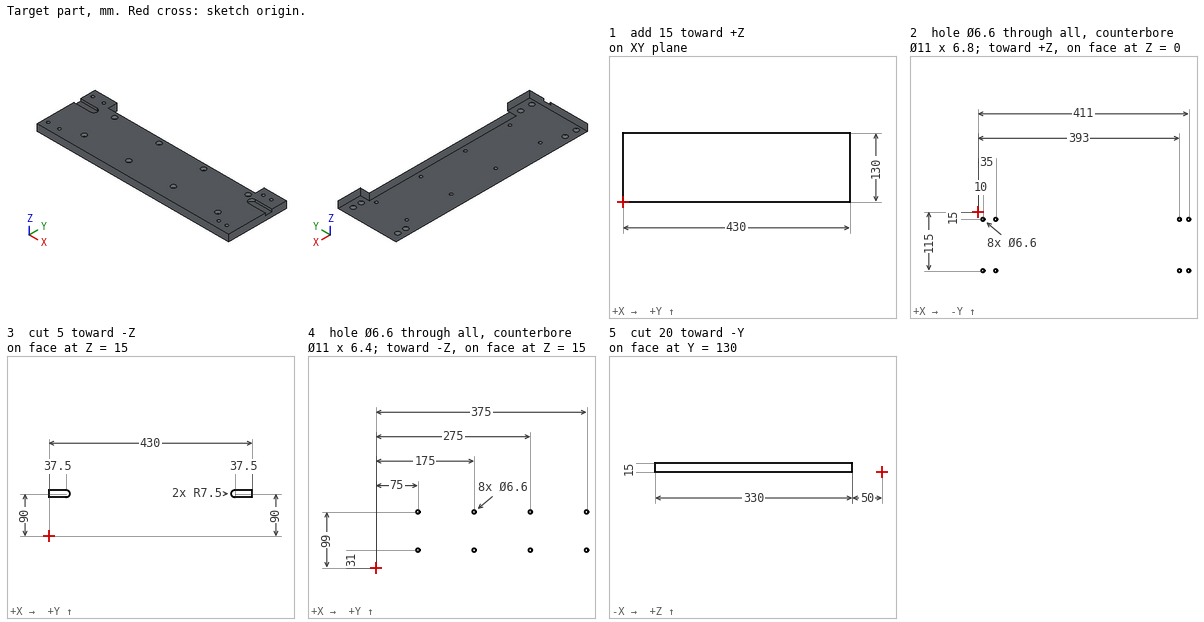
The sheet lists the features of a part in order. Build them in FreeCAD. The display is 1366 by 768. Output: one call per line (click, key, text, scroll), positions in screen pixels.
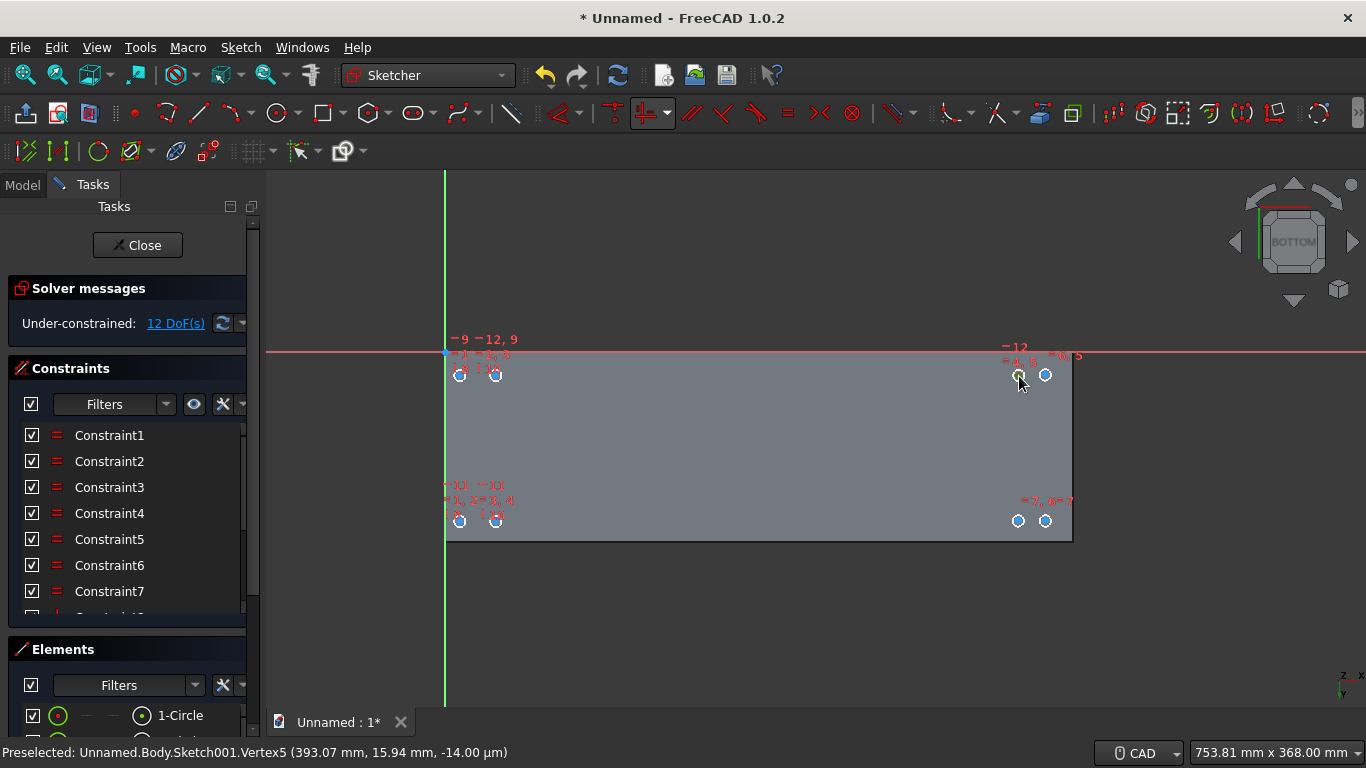
click(1045, 375)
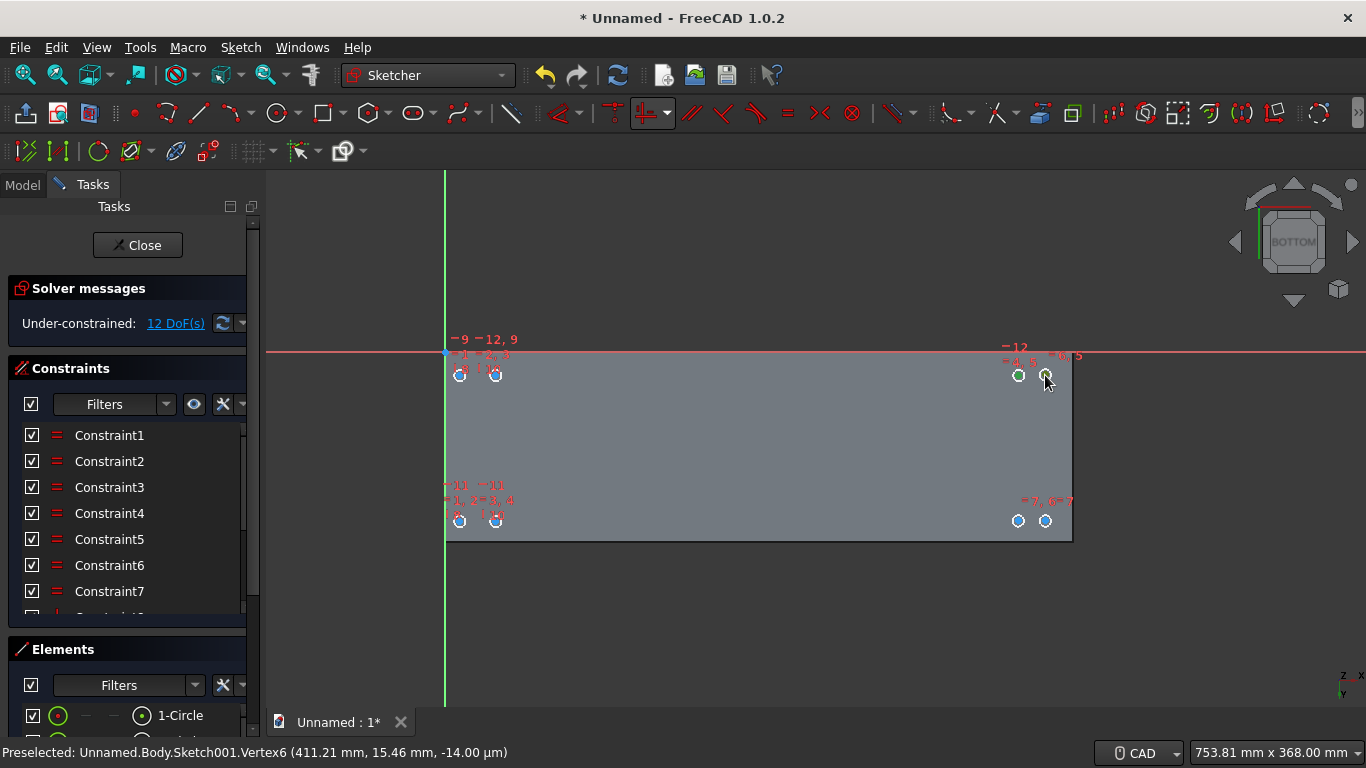
key(h)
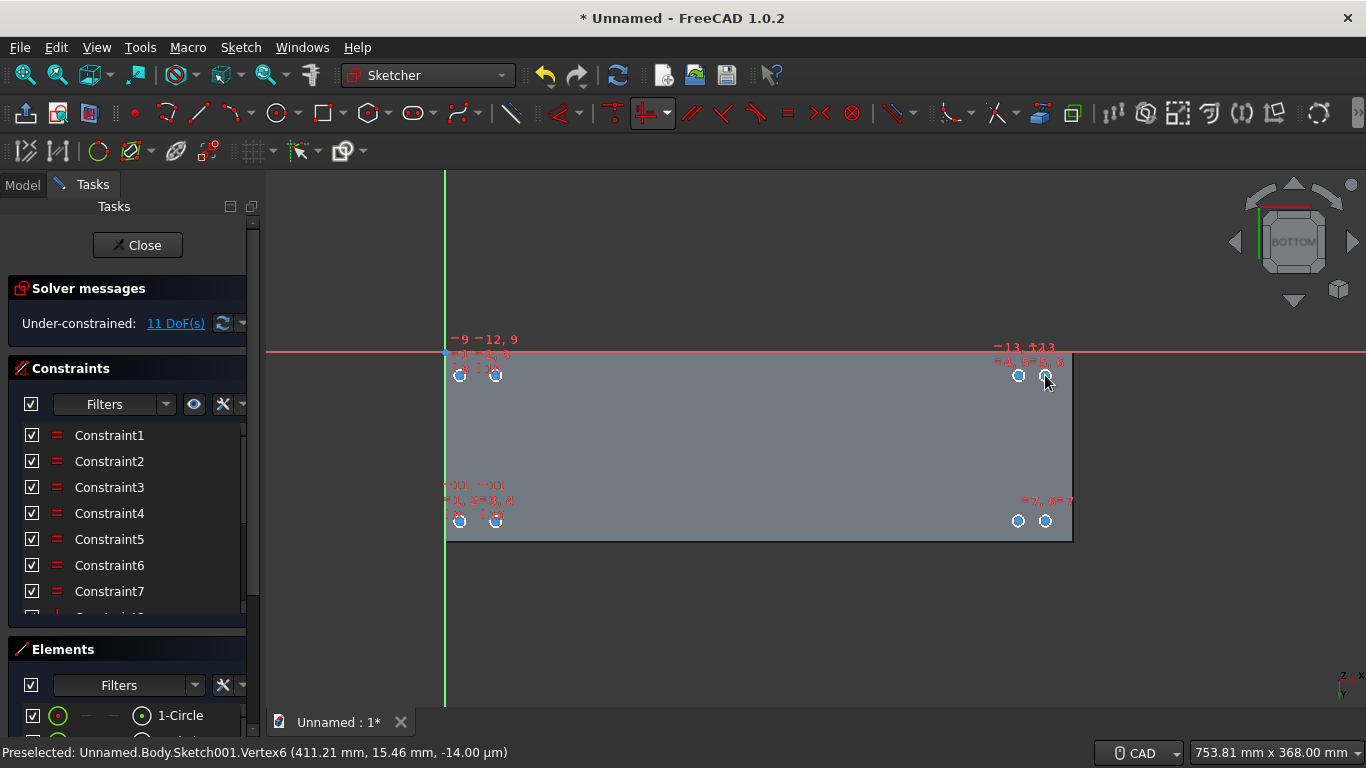
click(1019, 376)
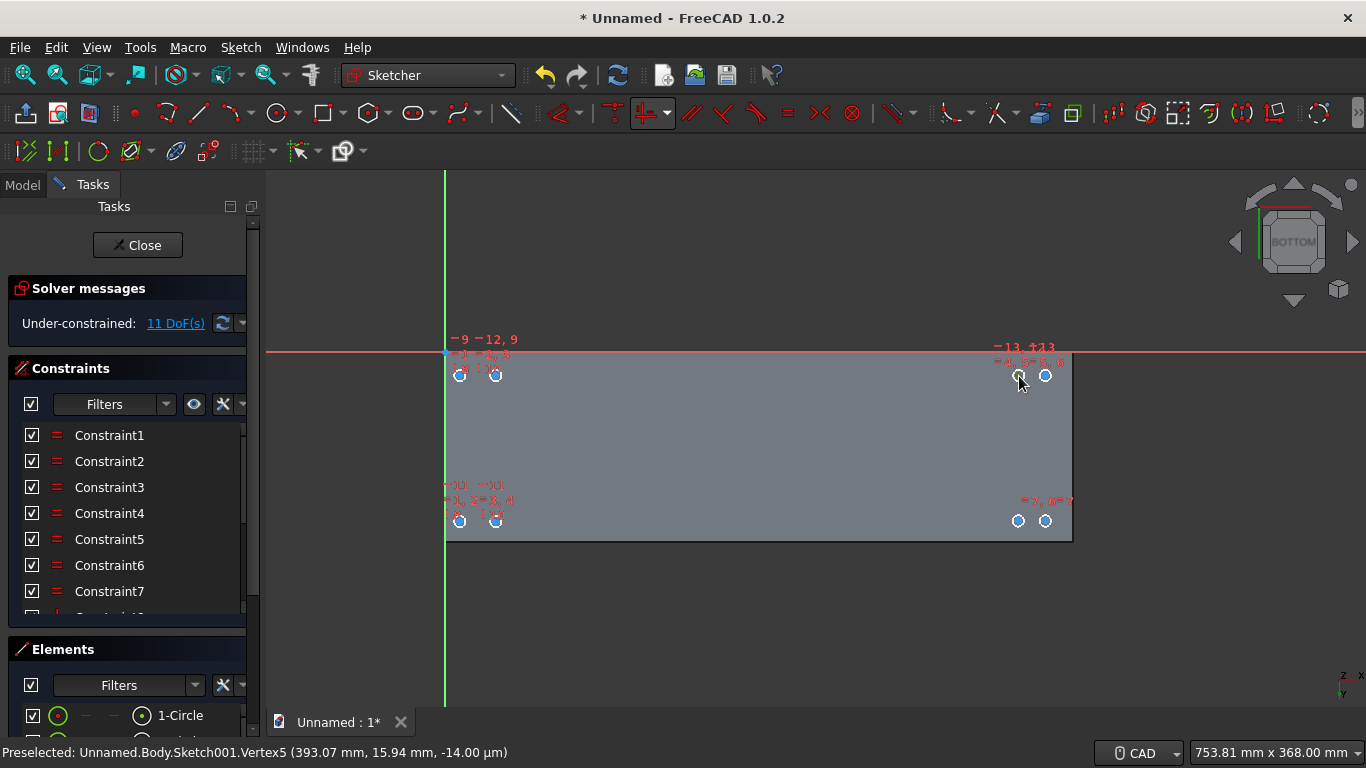
click(1018, 521)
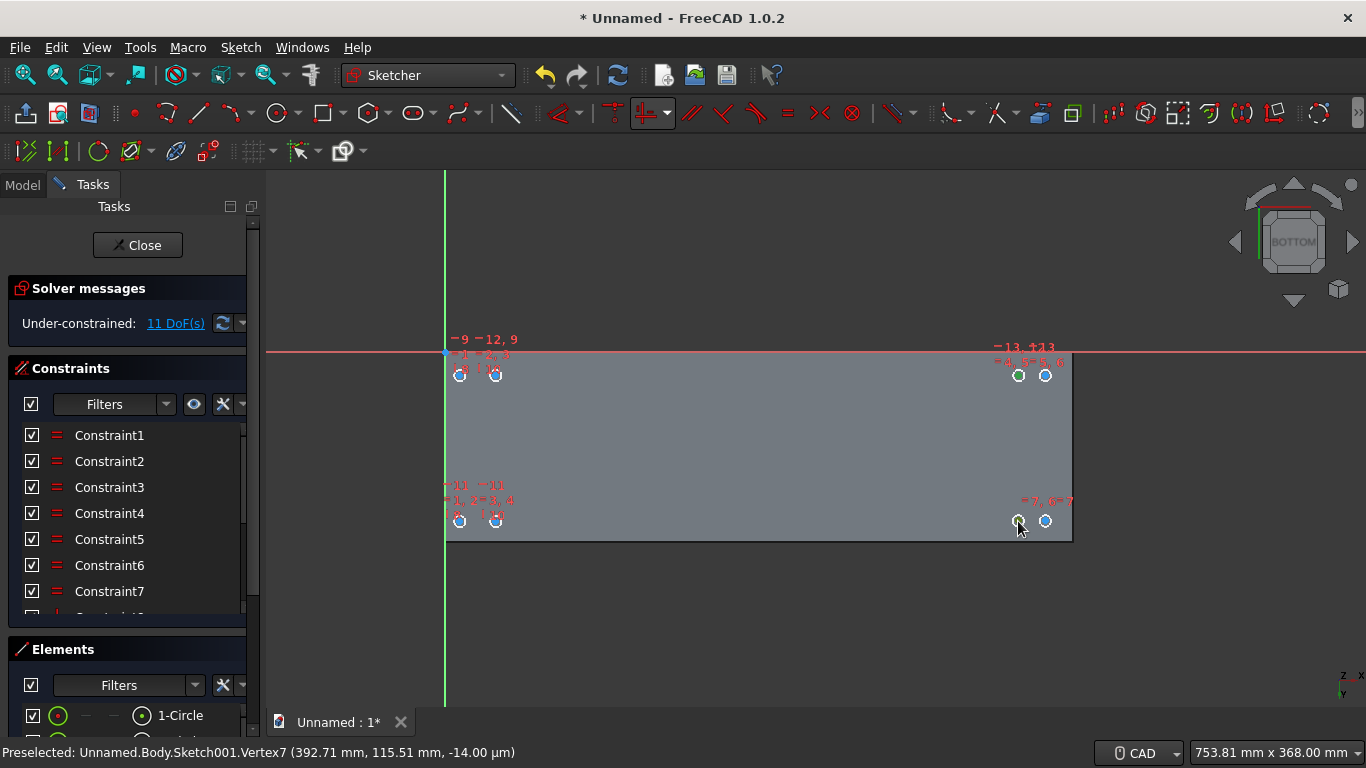
click(670, 114)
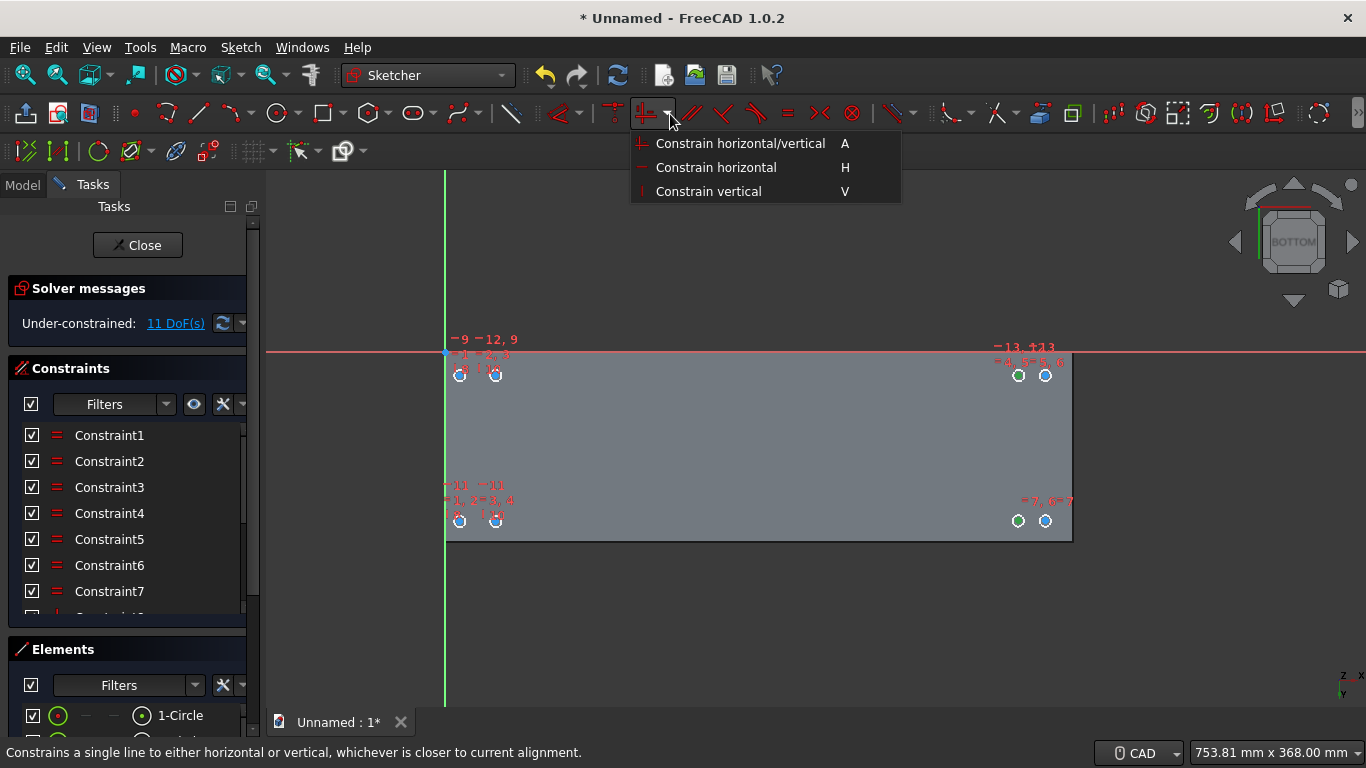
click(766, 191)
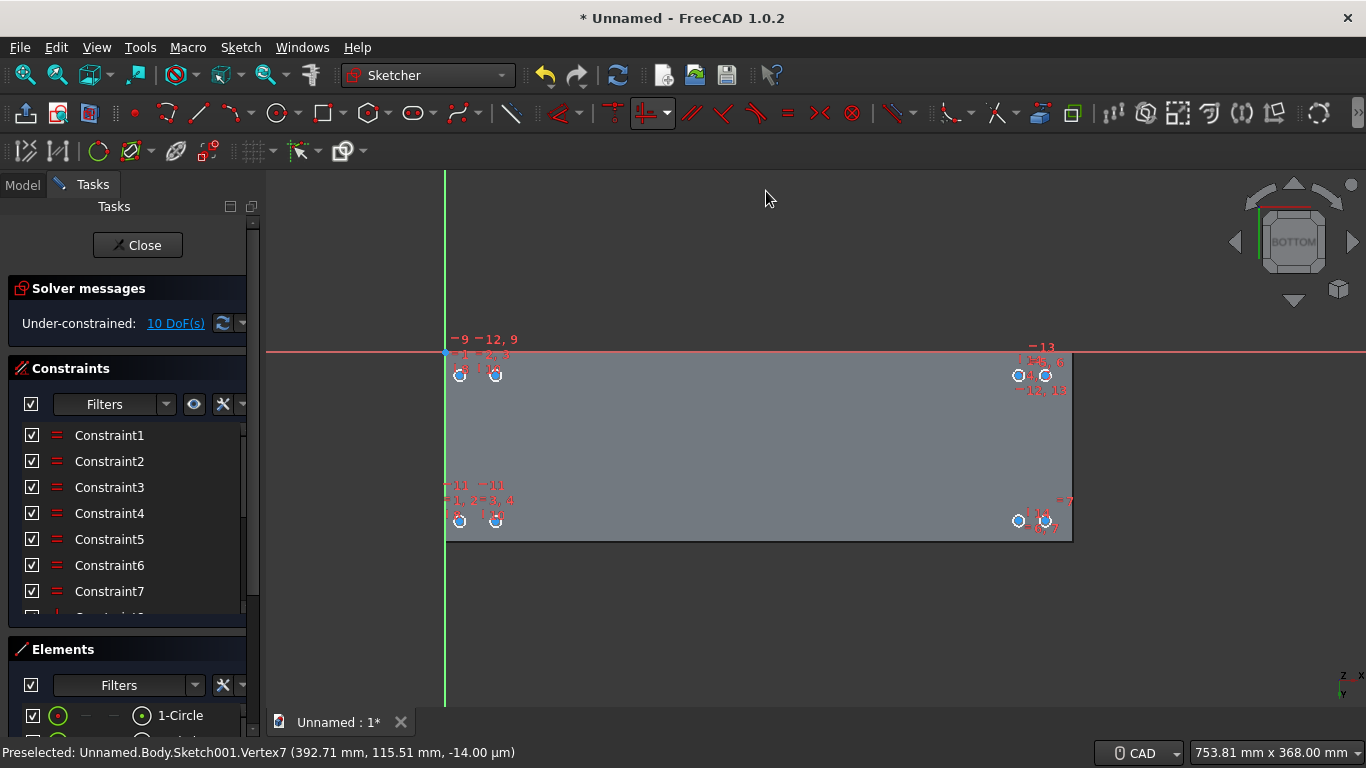
click(496, 522)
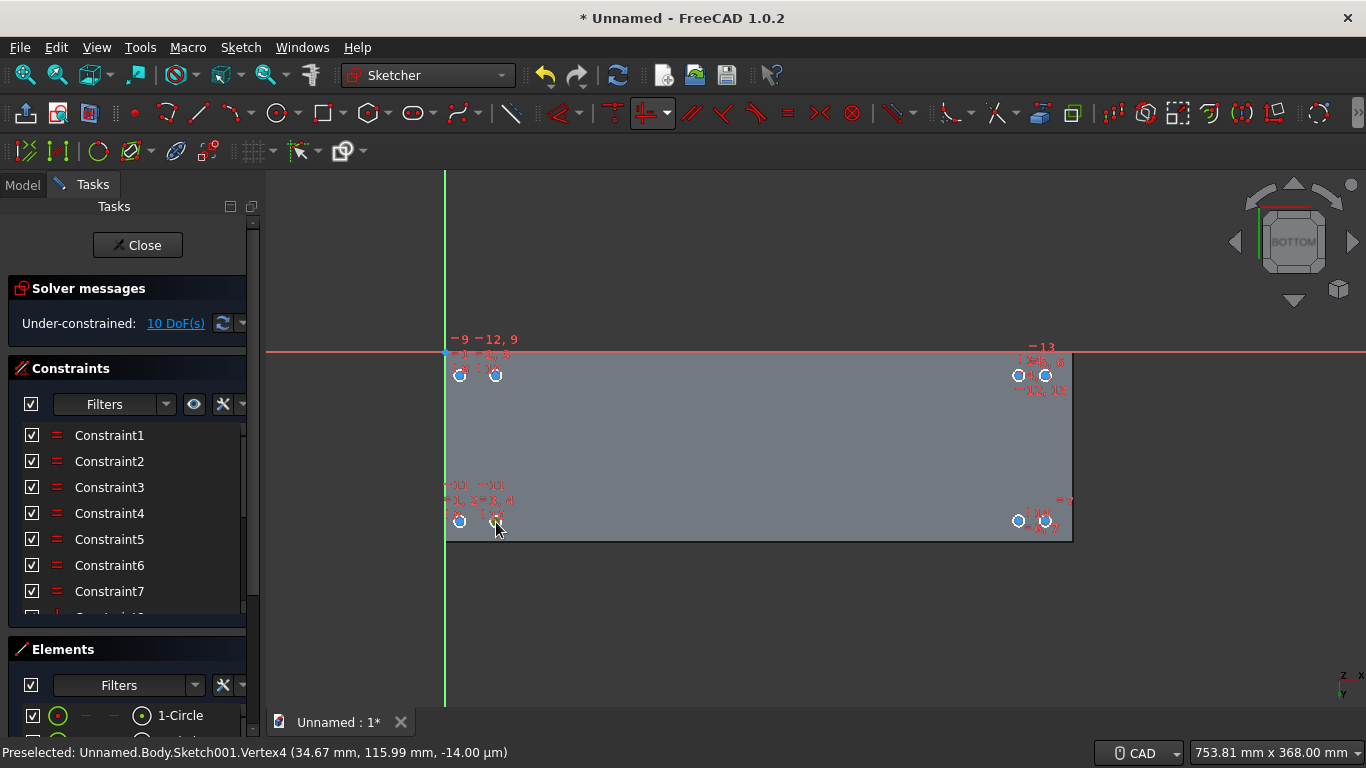
click(1019, 521)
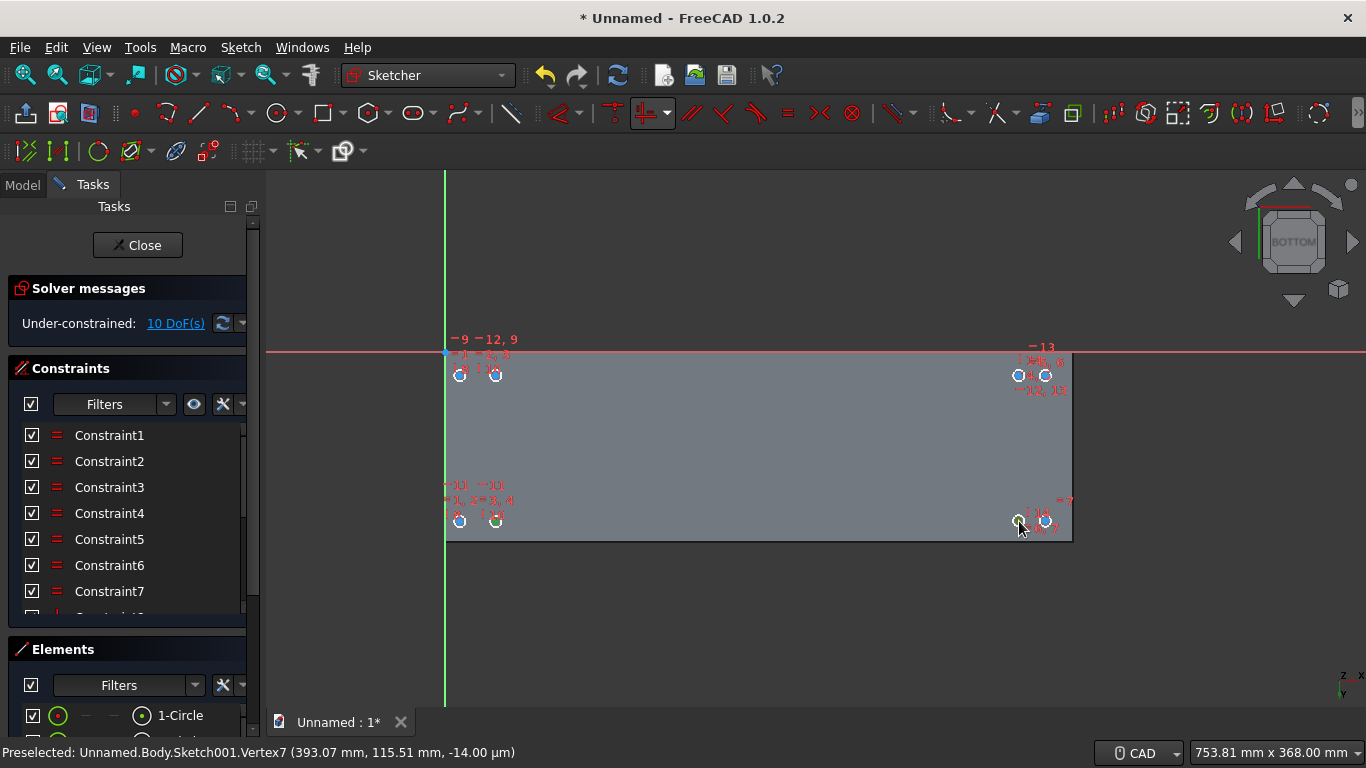
key(h)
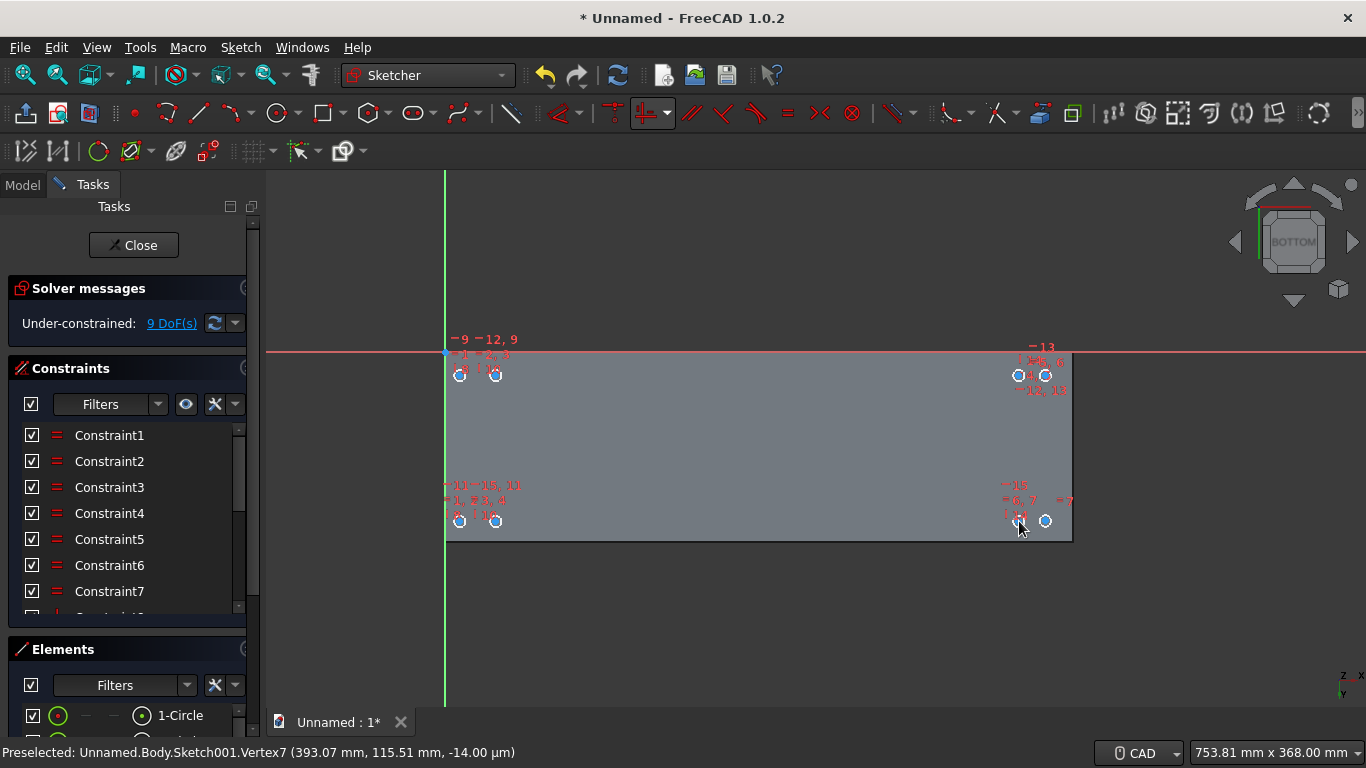
click(1045, 376)